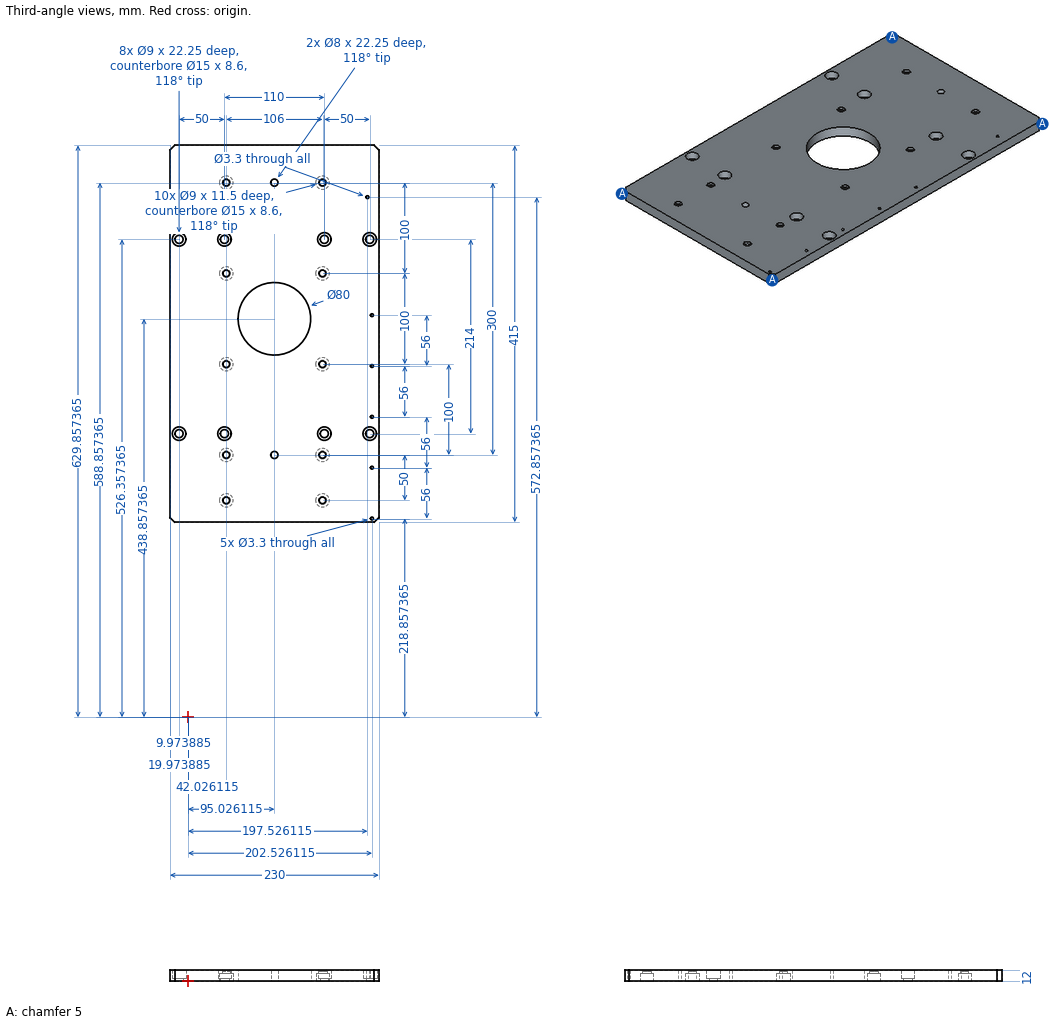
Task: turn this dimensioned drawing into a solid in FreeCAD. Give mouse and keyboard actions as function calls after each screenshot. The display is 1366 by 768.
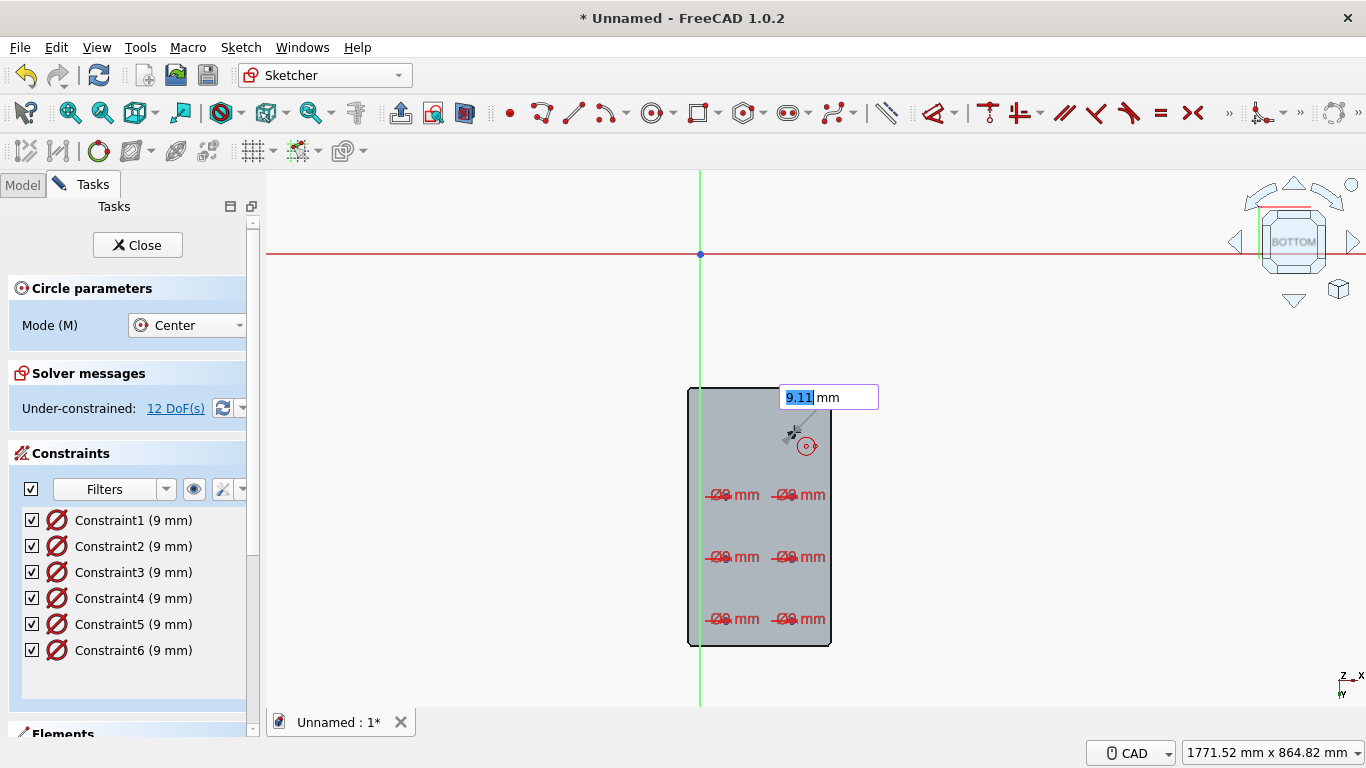
text(9)
key(Return)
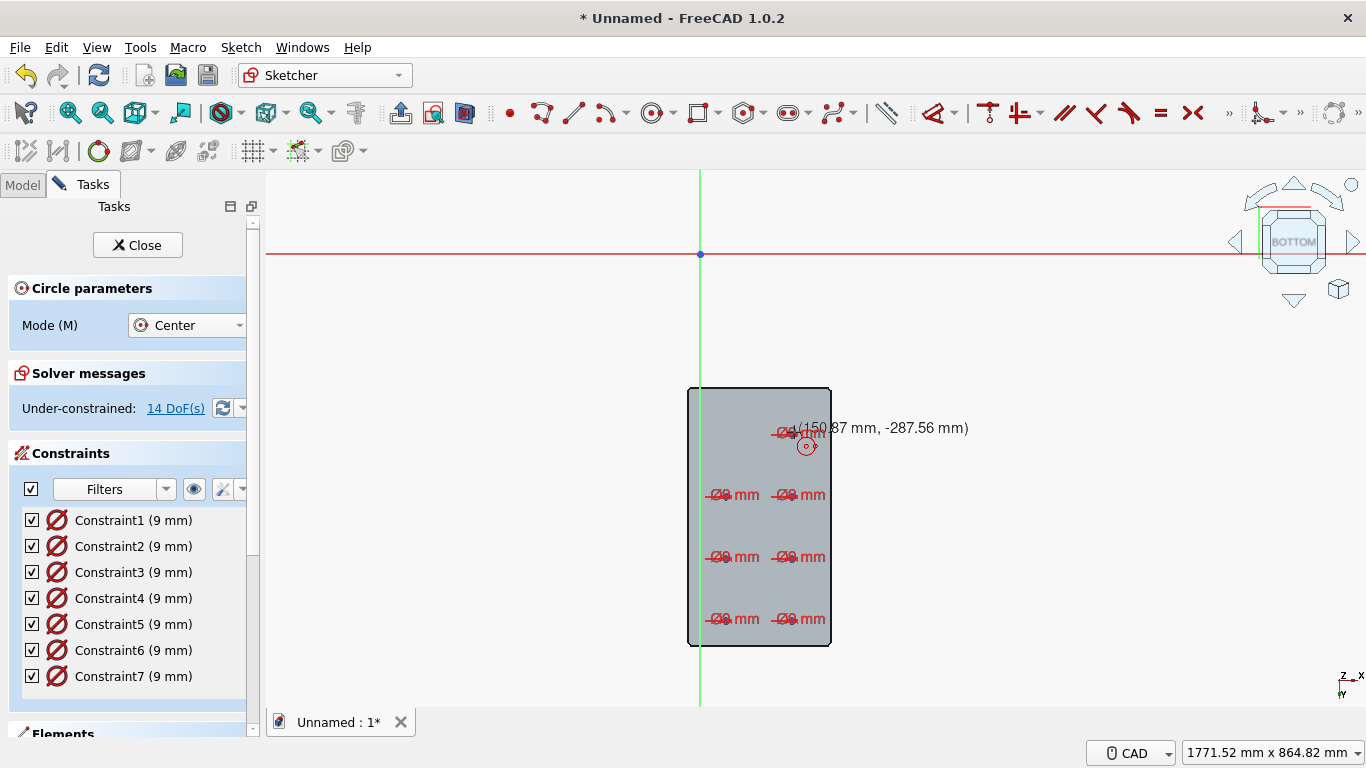
scroll(726, 434, up, 11)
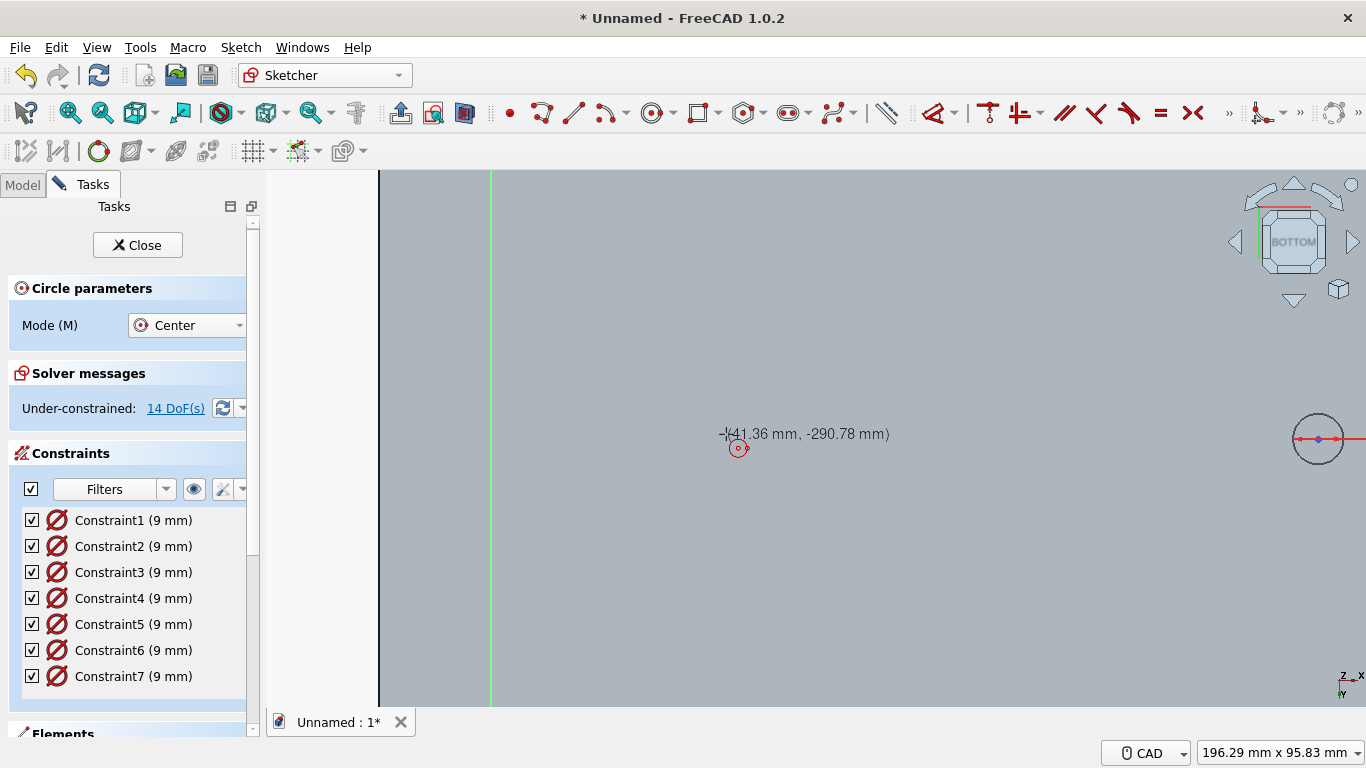
scroll(726, 434, down, 11)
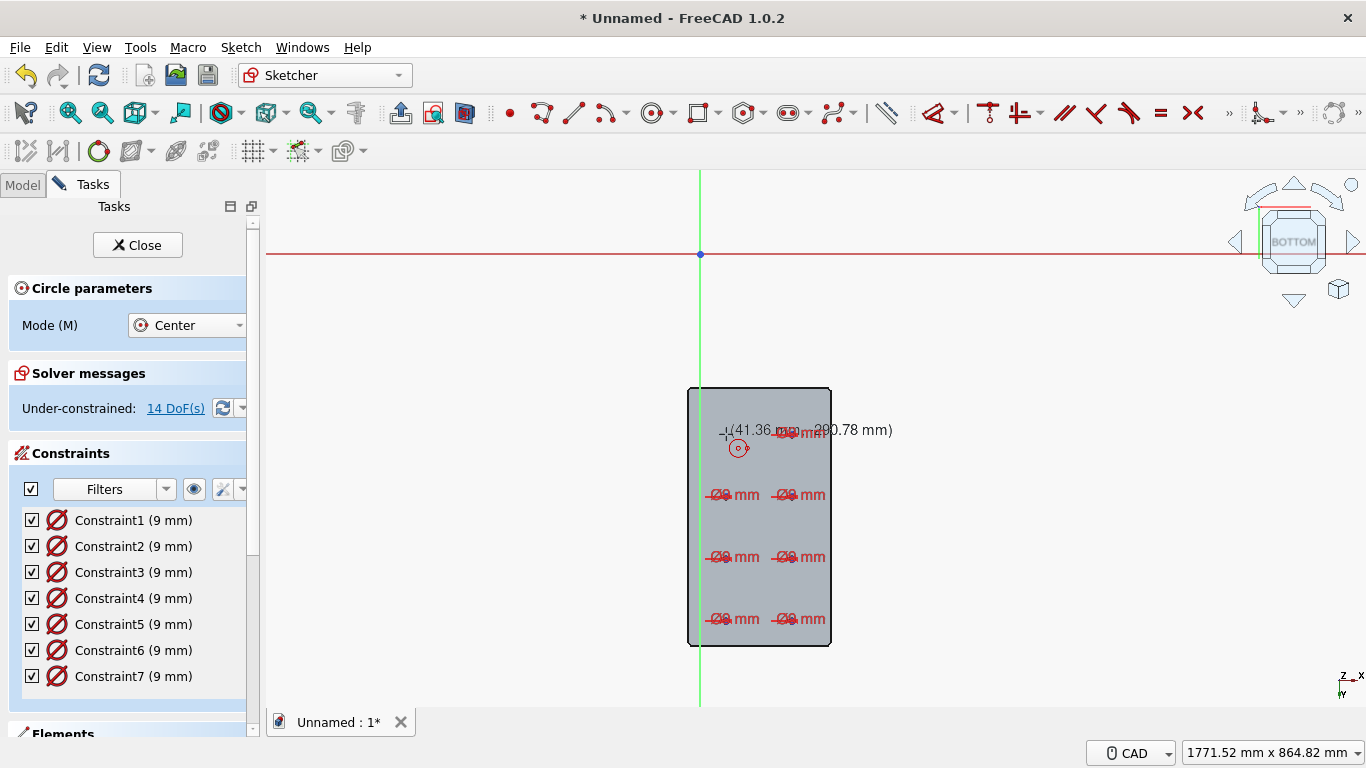
click(726, 434)
move(728, 432)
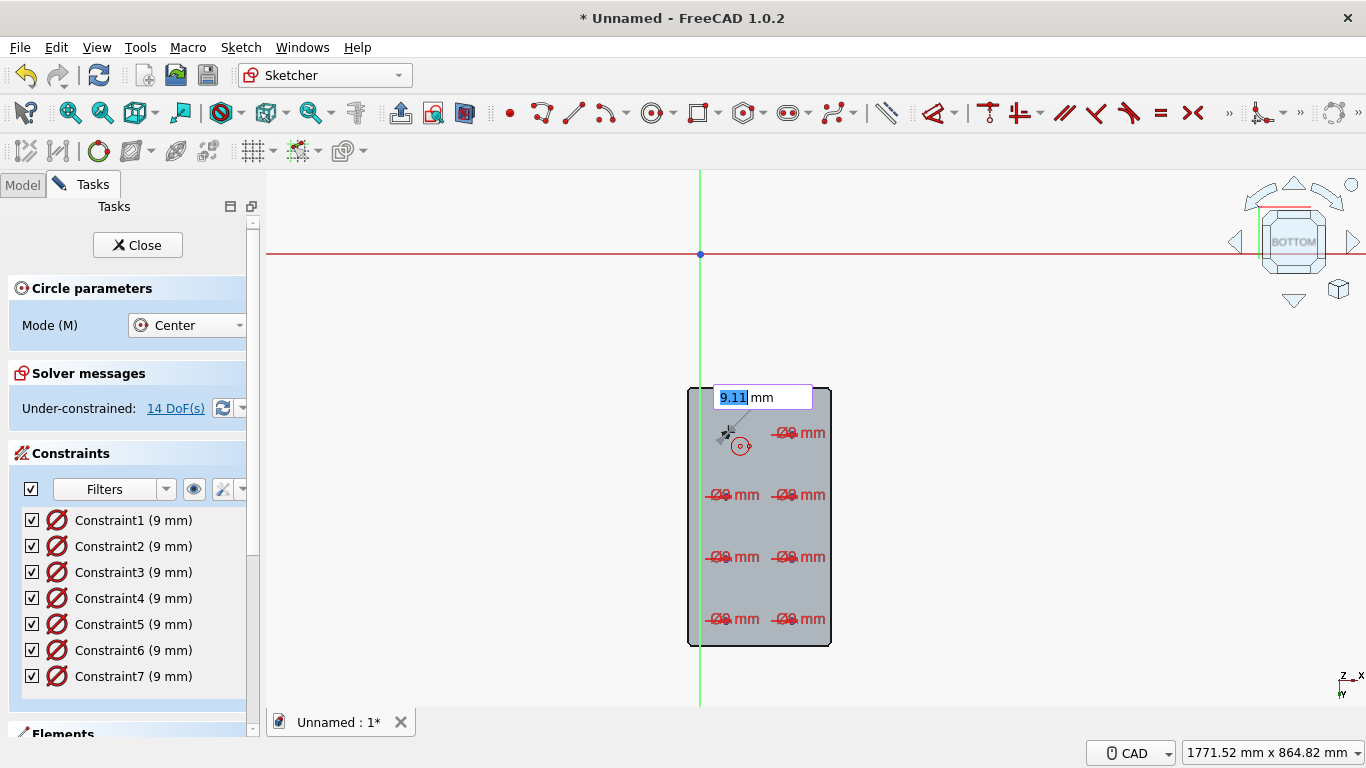
text(9)
key(Return)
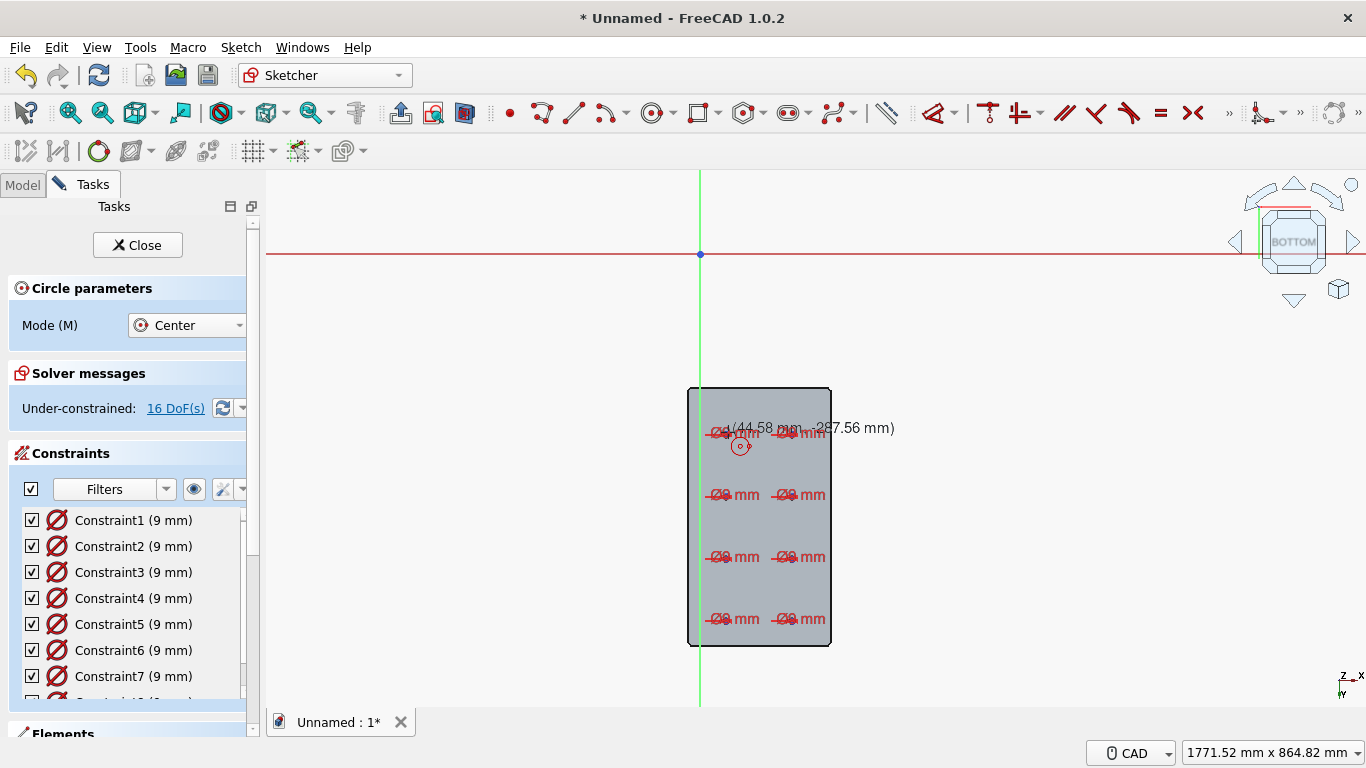
scroll(792, 403, up, 11)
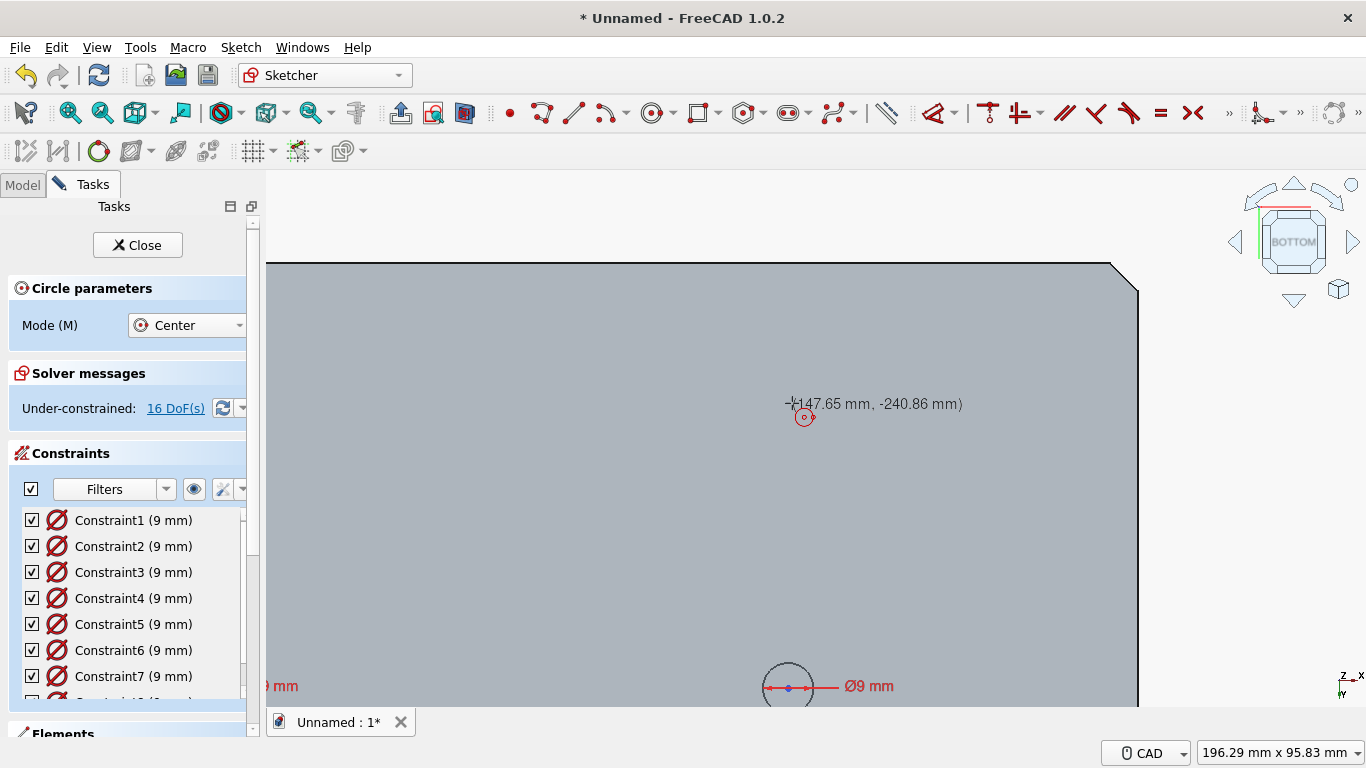
scroll(792, 403, down, 11)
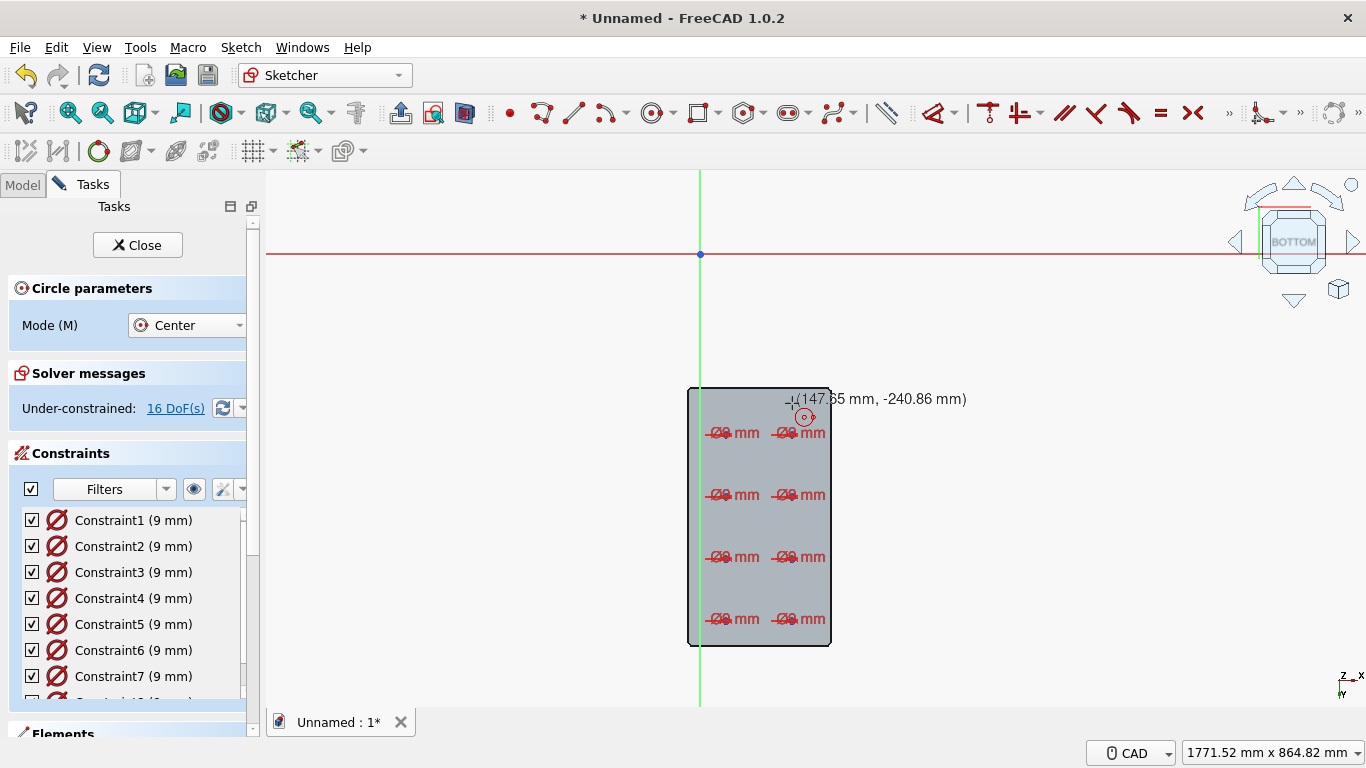
click(792, 403)
move(794, 401)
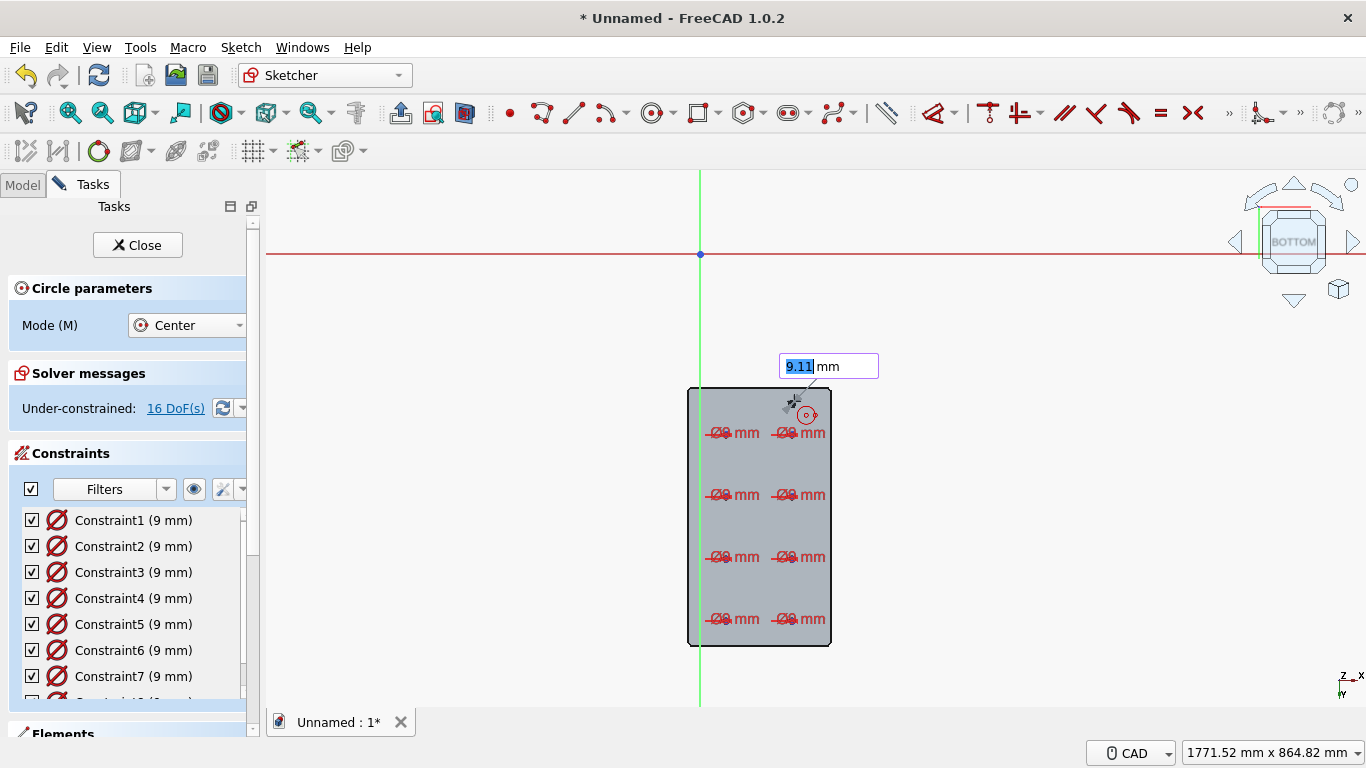
text(9)
key(Return)